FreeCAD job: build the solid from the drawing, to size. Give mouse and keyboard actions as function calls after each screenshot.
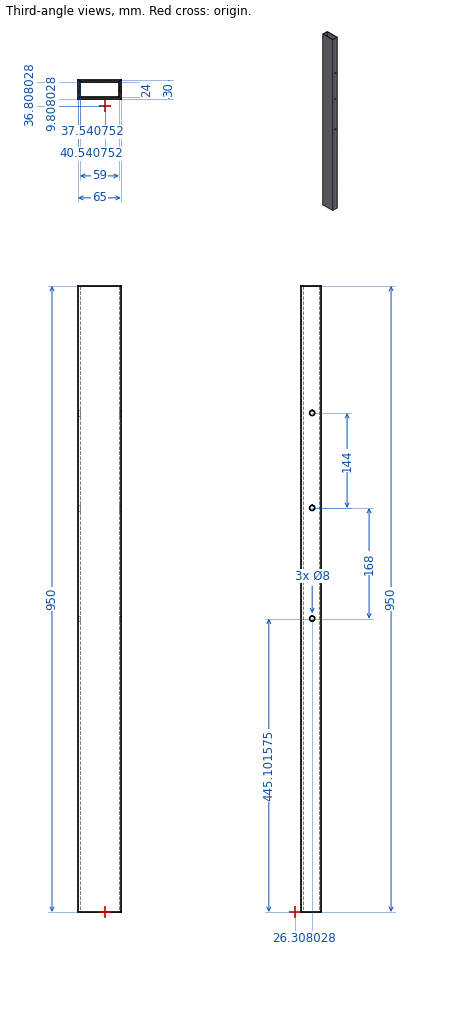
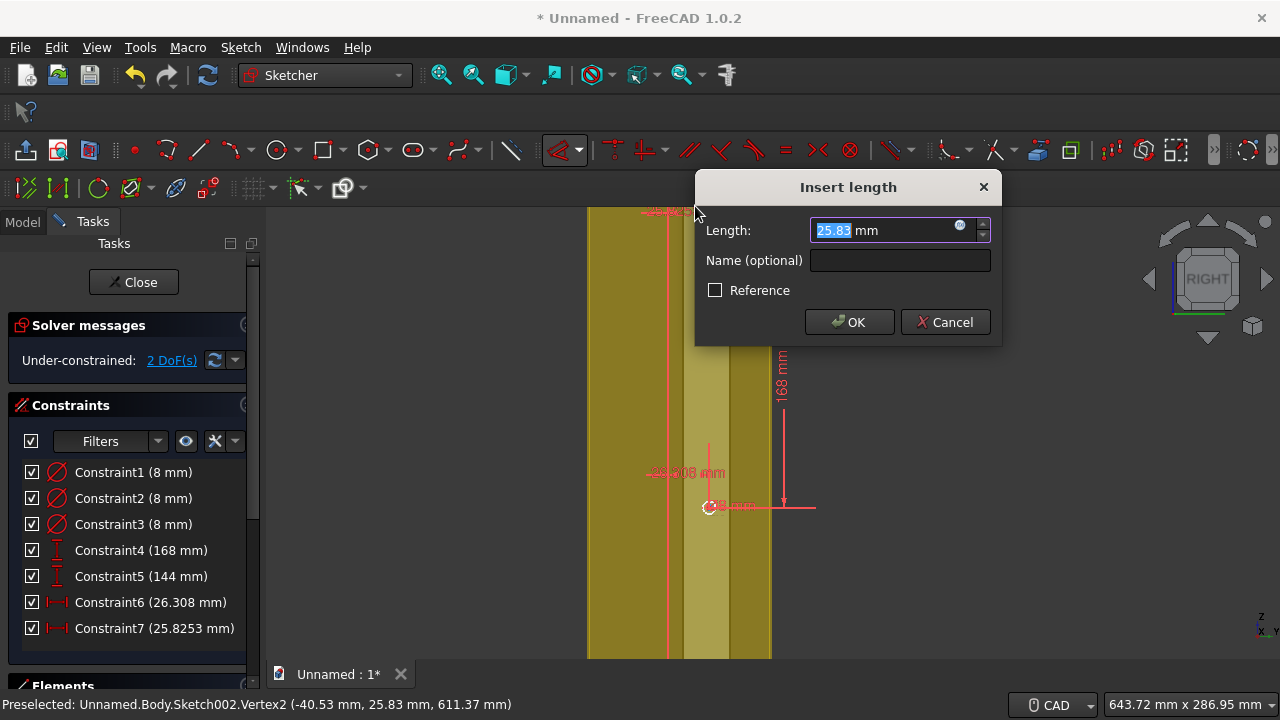
text(26.308028)
key(Return)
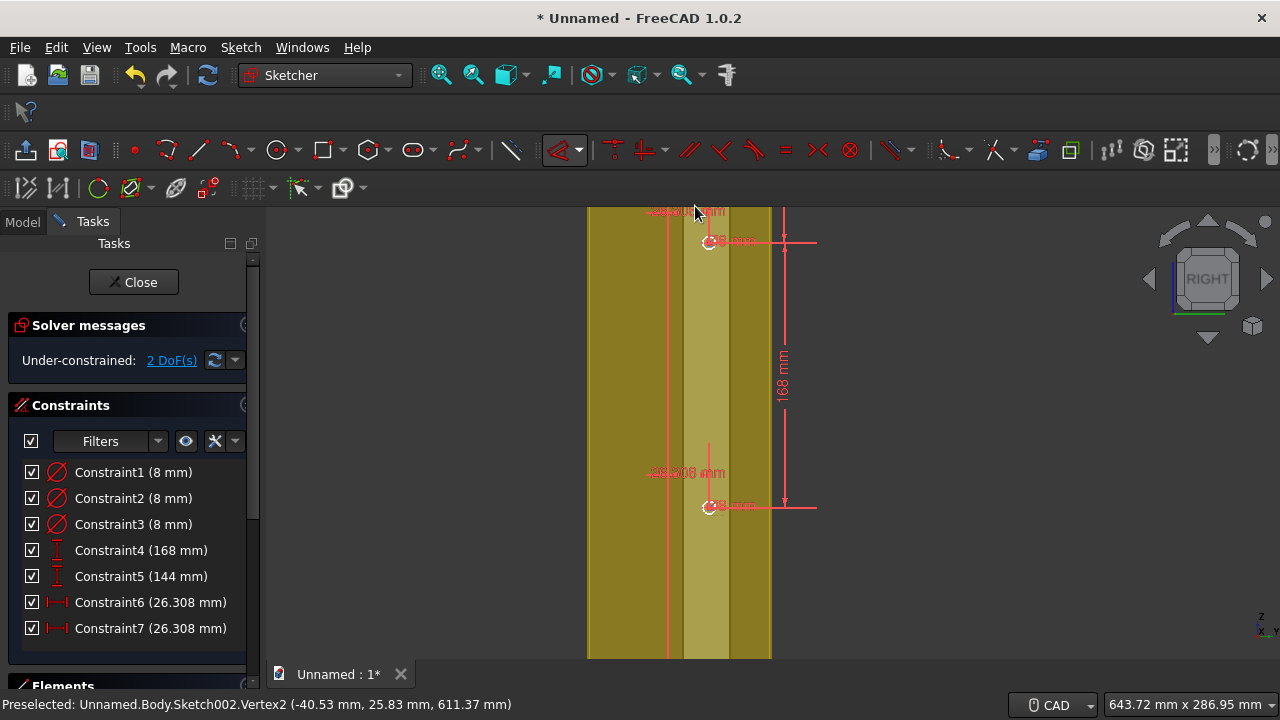
scroll(709, 376, down, 7)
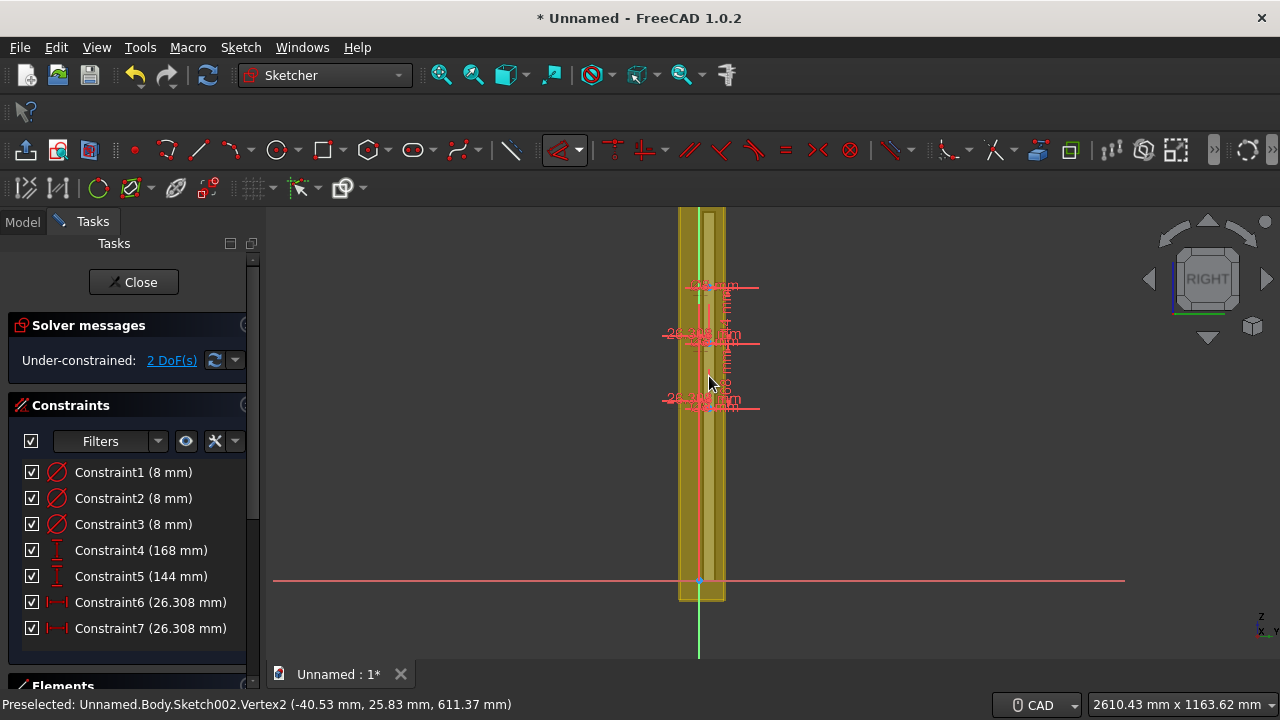
scroll(709, 288, up, 7)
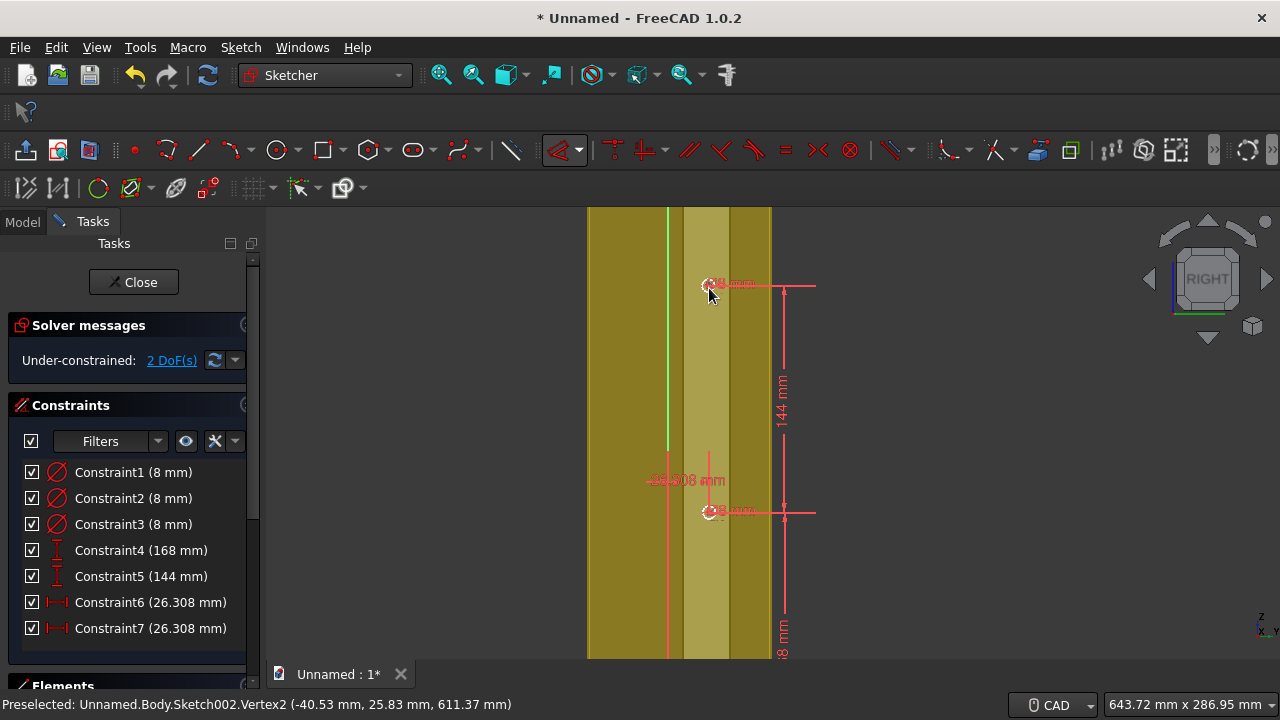
click(708, 286)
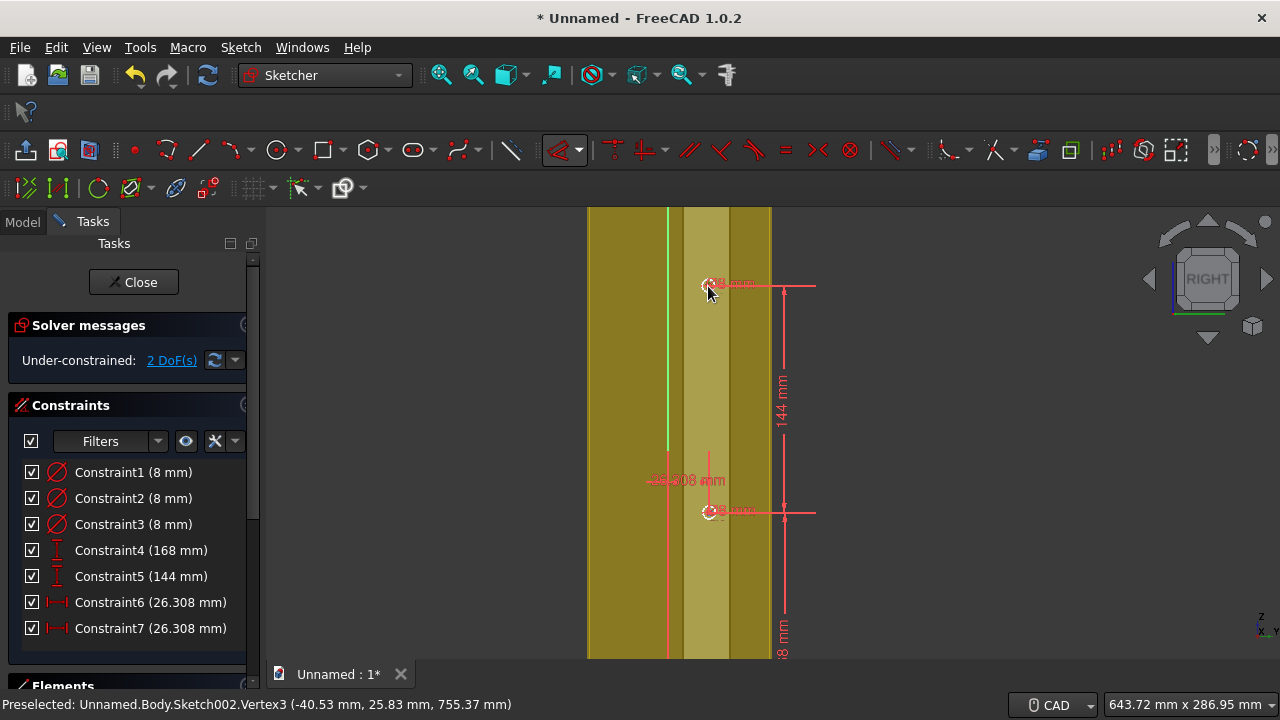
click(582, 150)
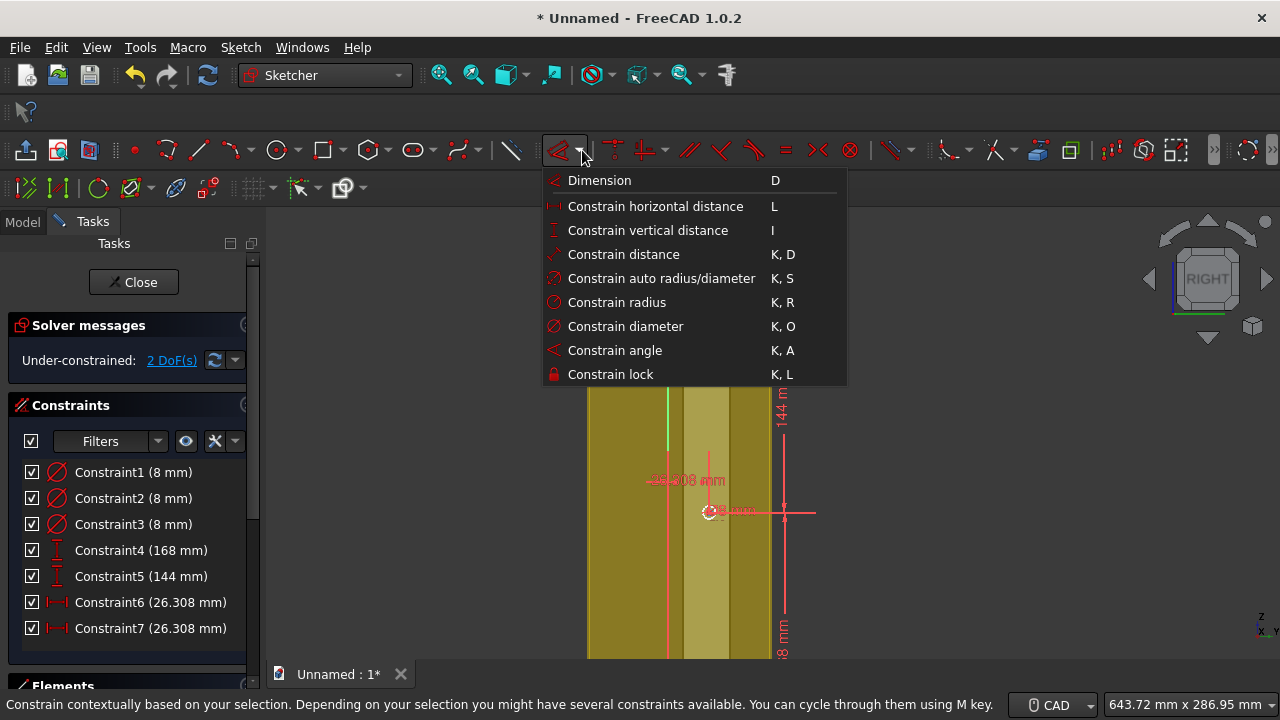
click(695, 206)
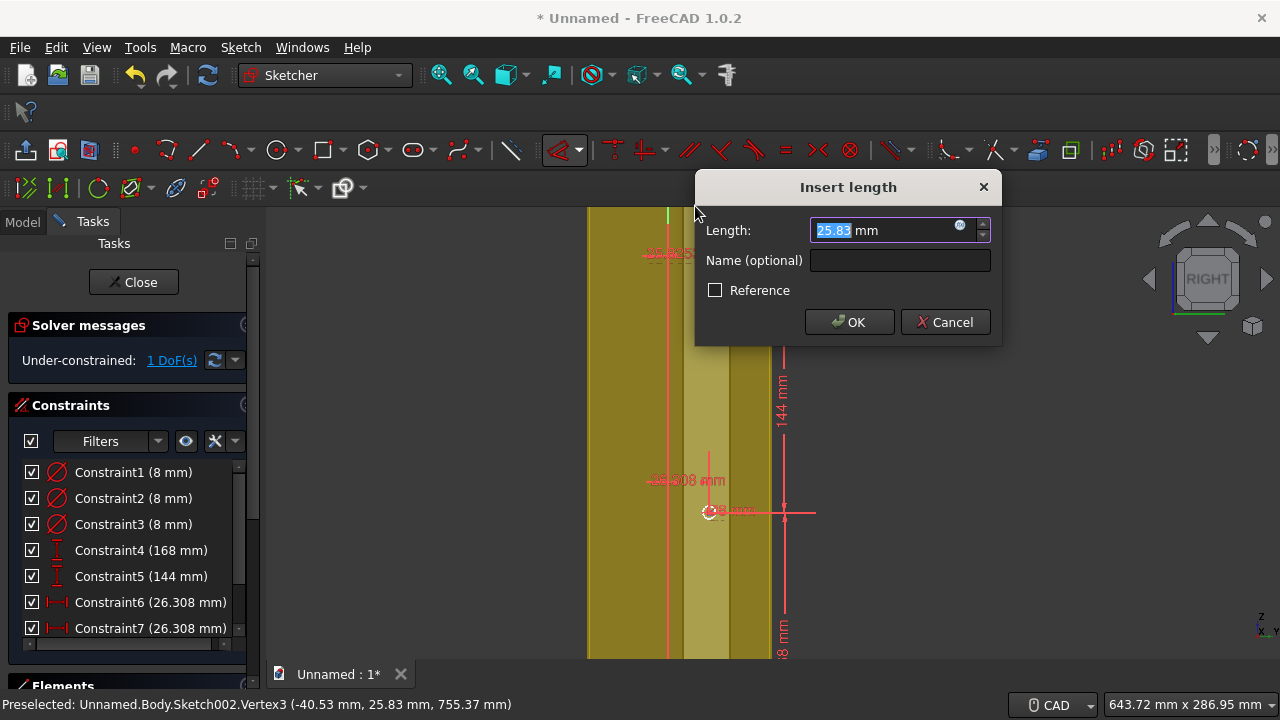
text(26.308028)
key(Return)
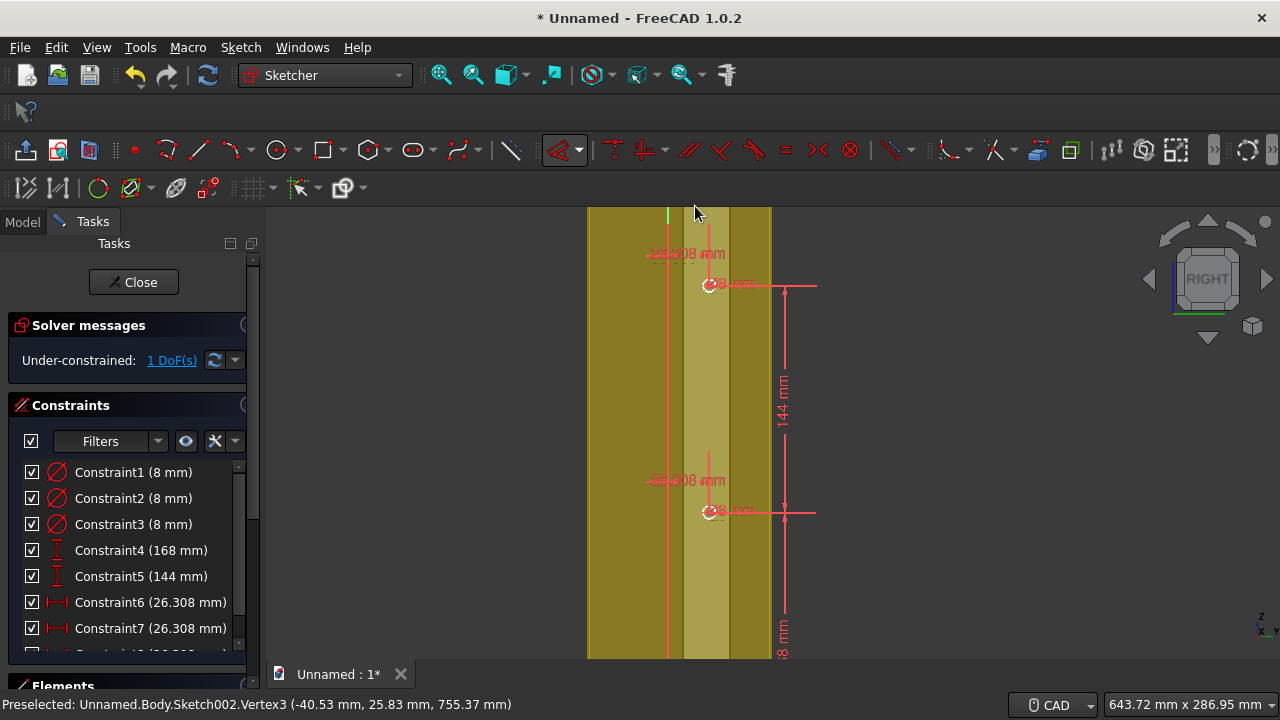
scroll(709, 288, down, 7)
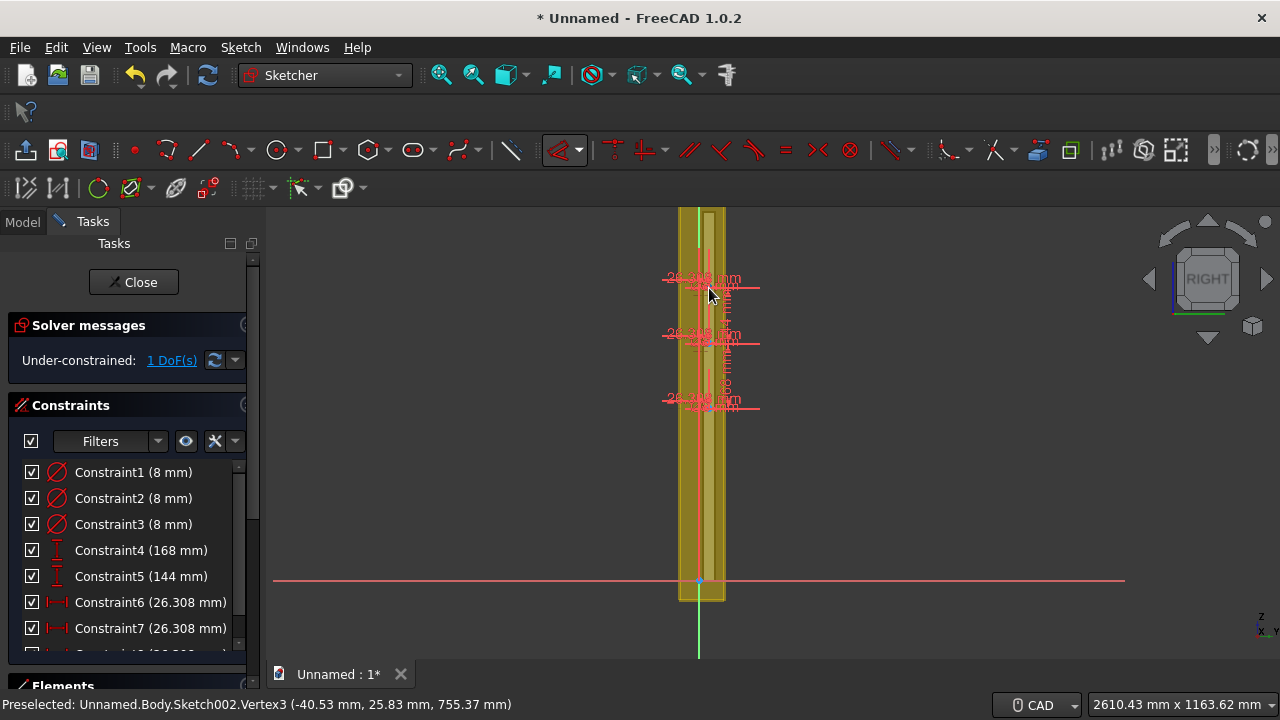
click(709, 409)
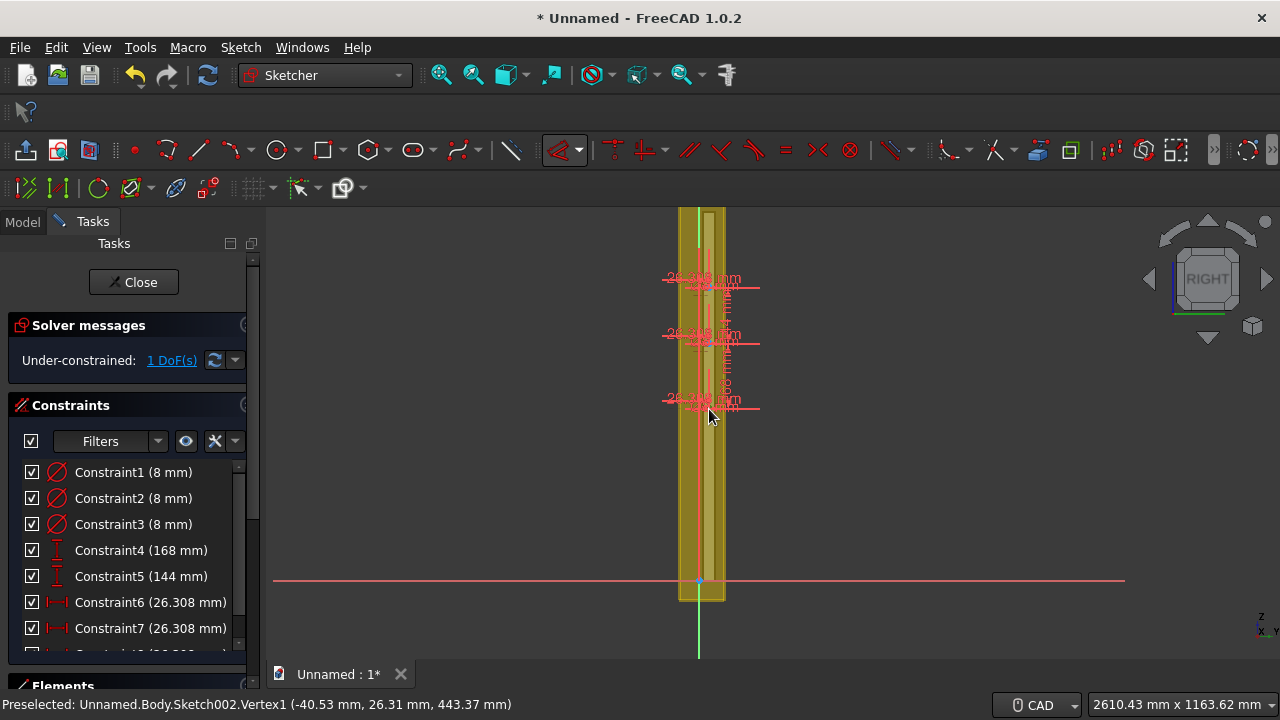
key(i)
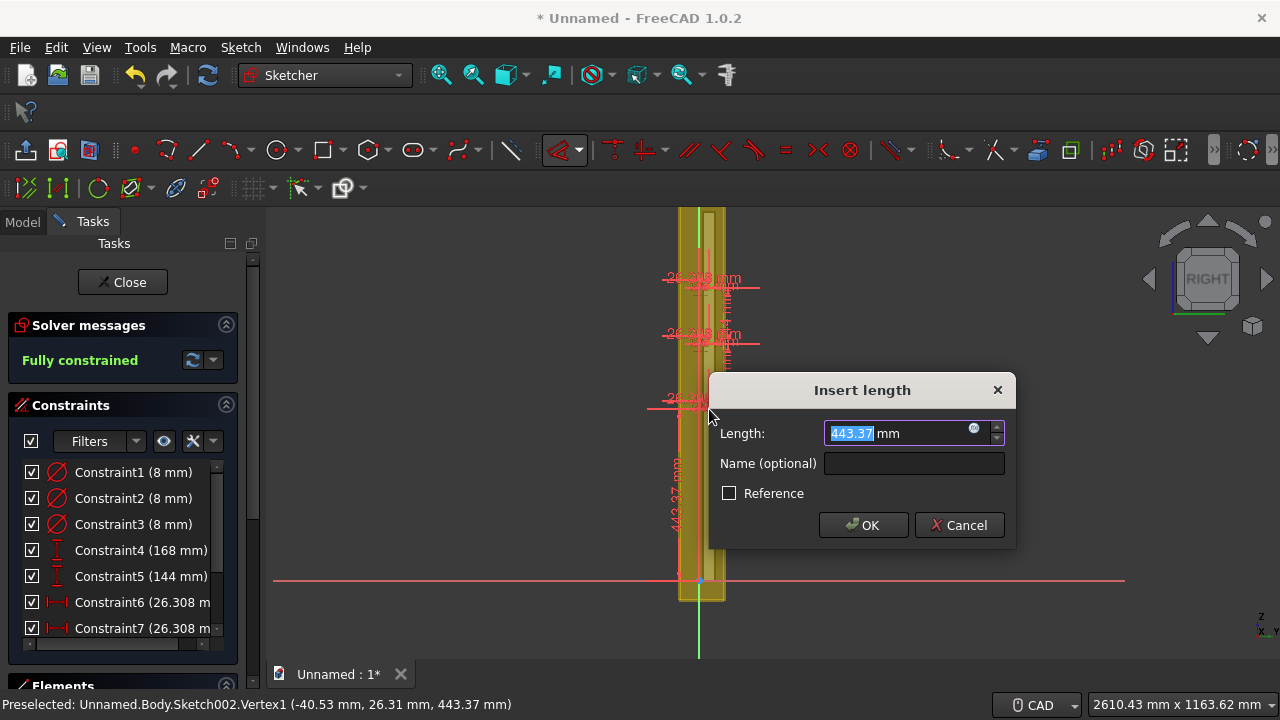
text(445.101575)
key(Return)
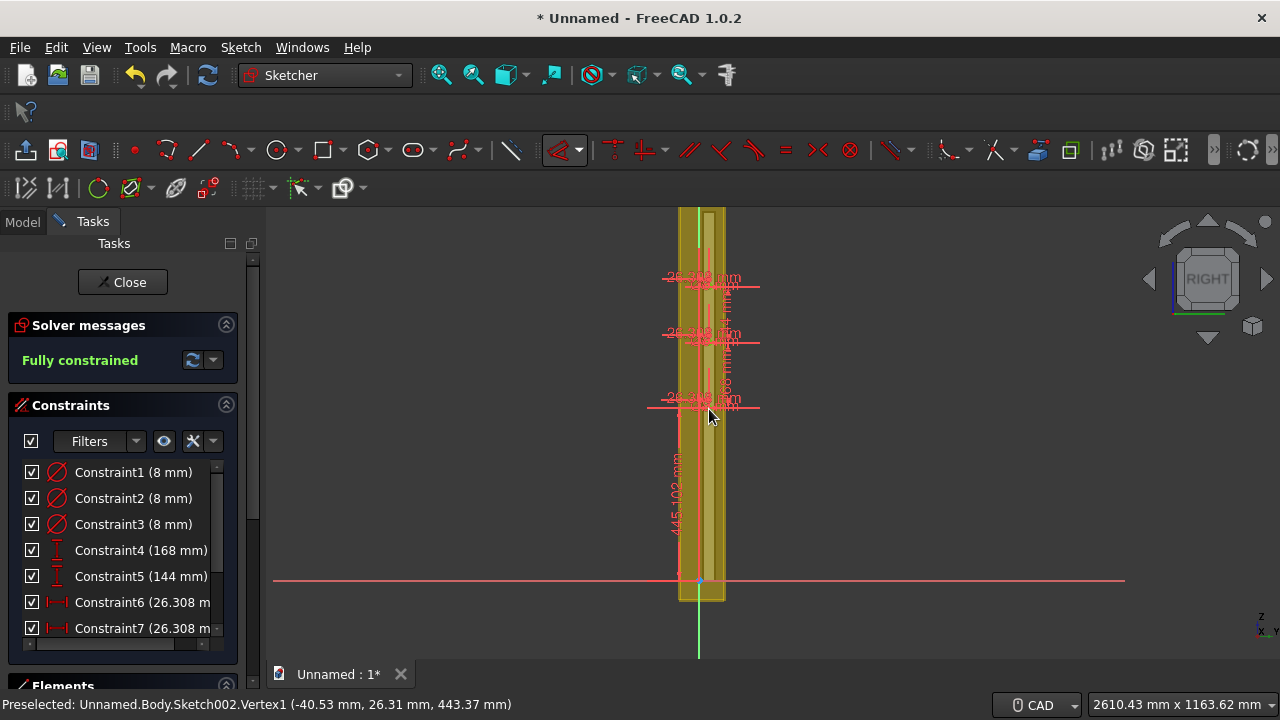
click(123, 282)